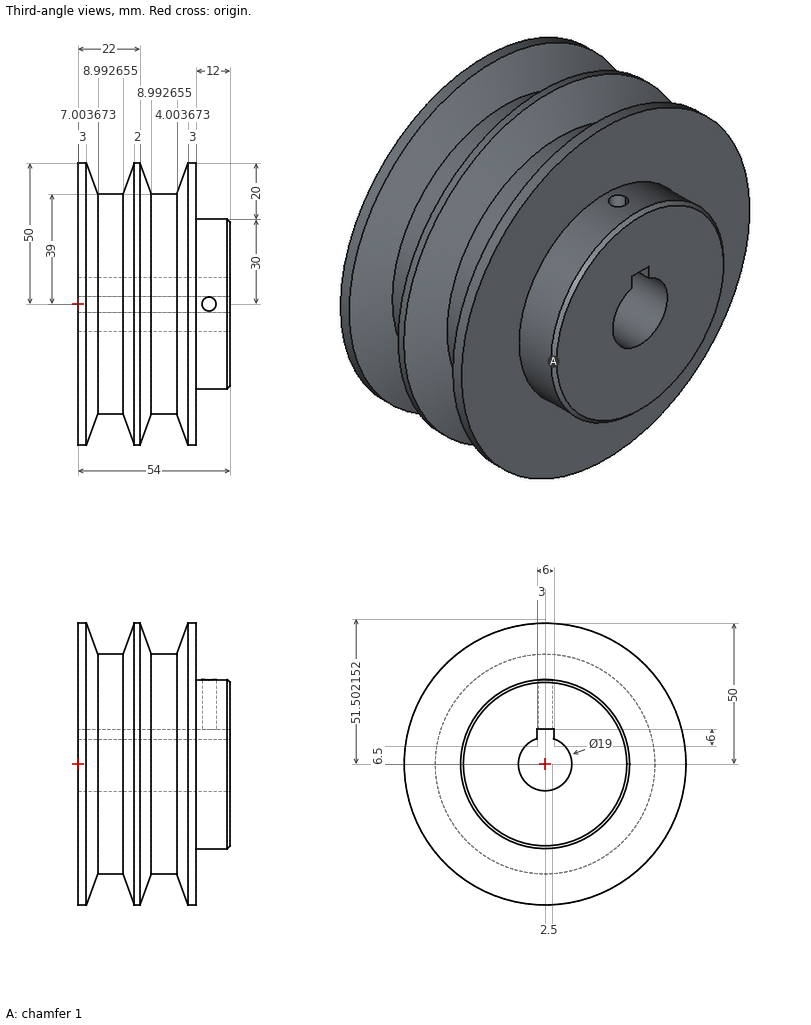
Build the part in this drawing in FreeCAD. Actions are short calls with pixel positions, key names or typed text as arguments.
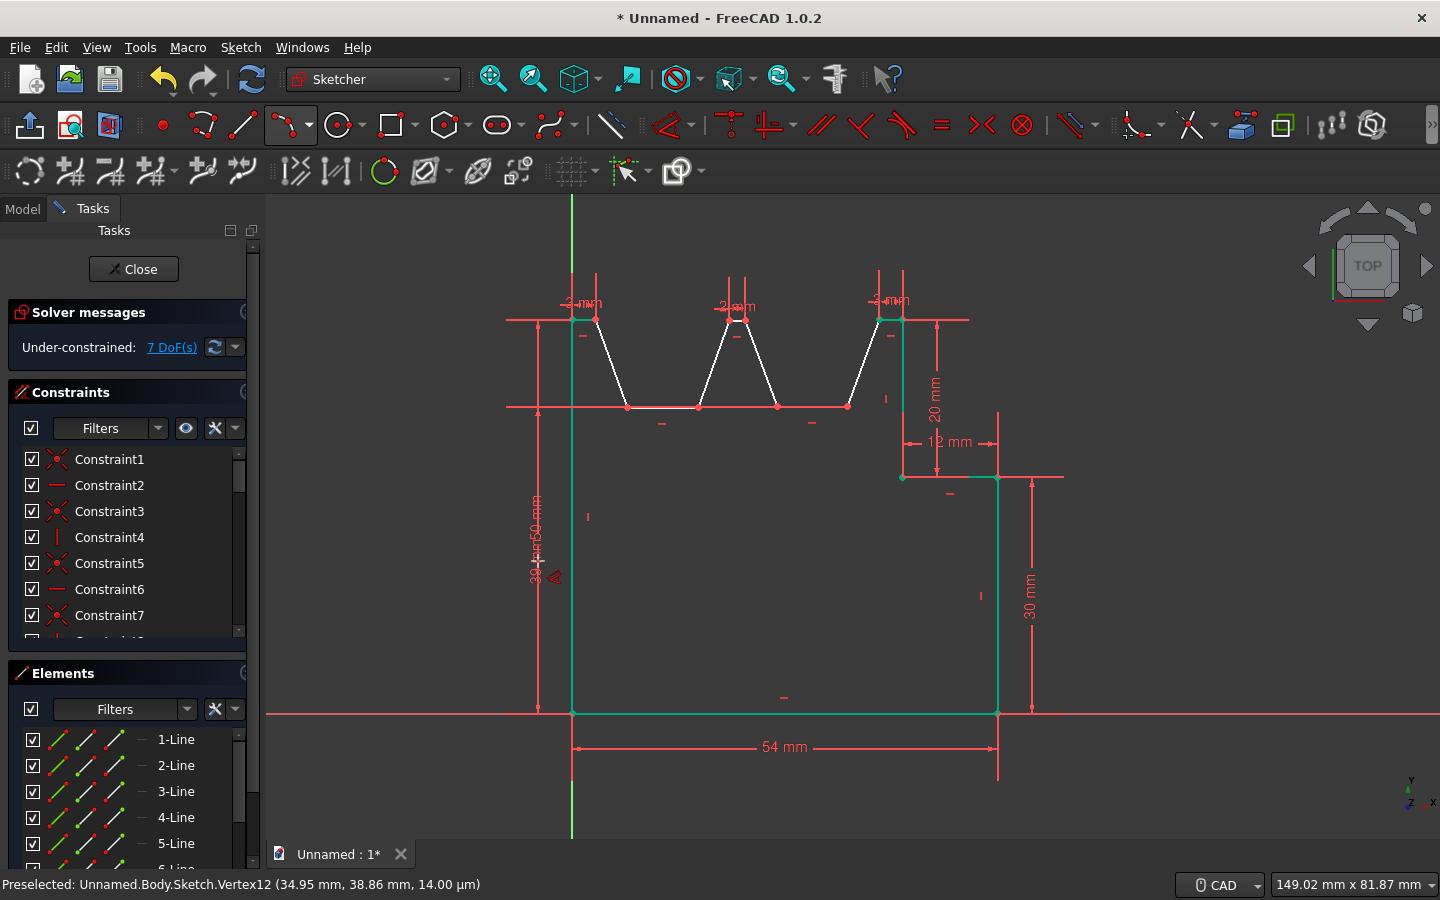
click(745, 321)
click(659, 748)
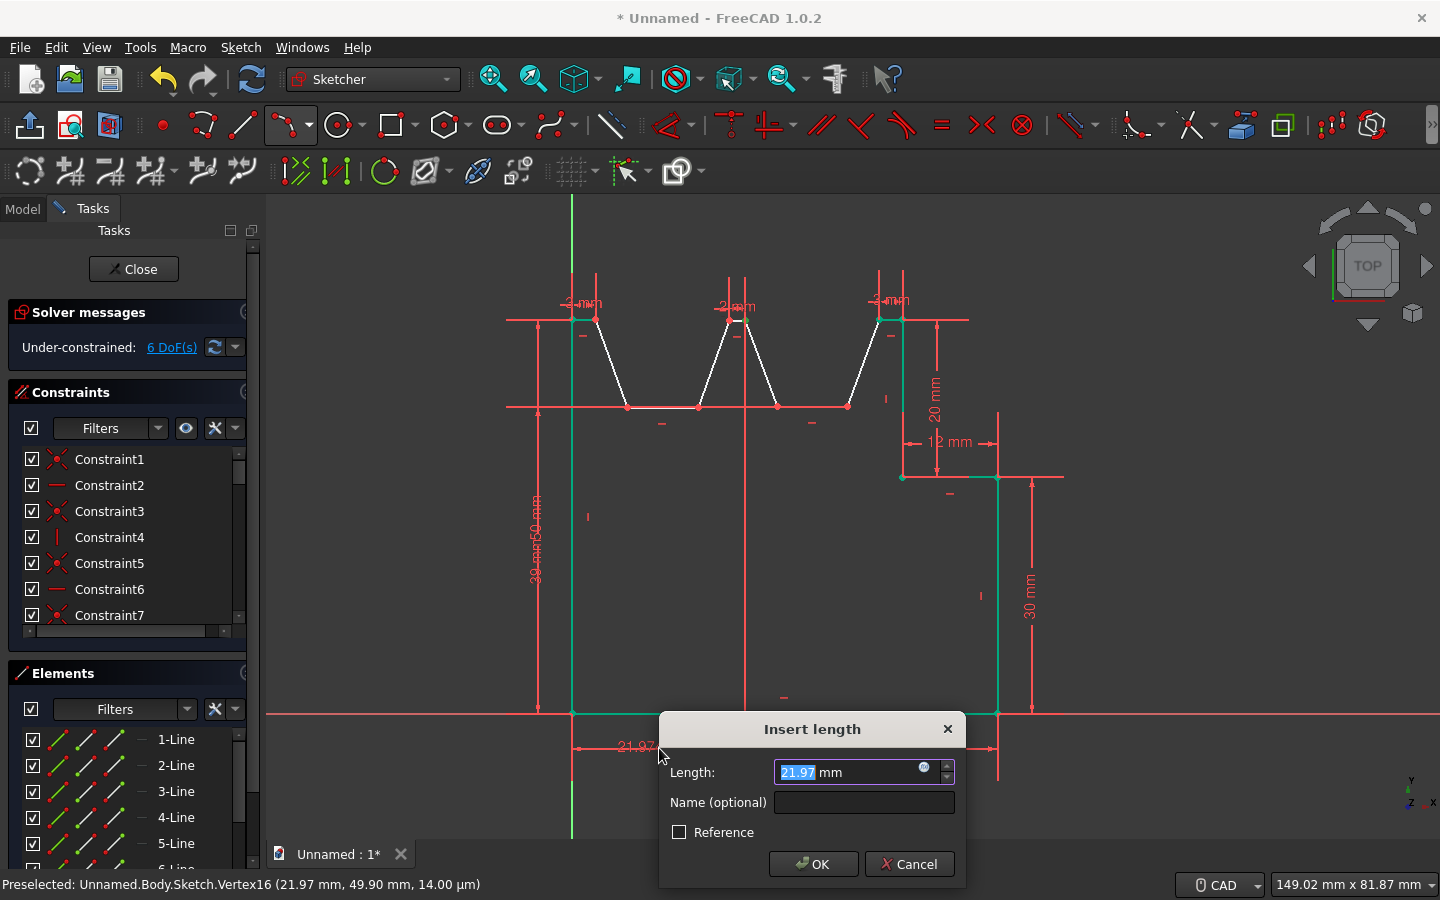
text(22)
key(Return)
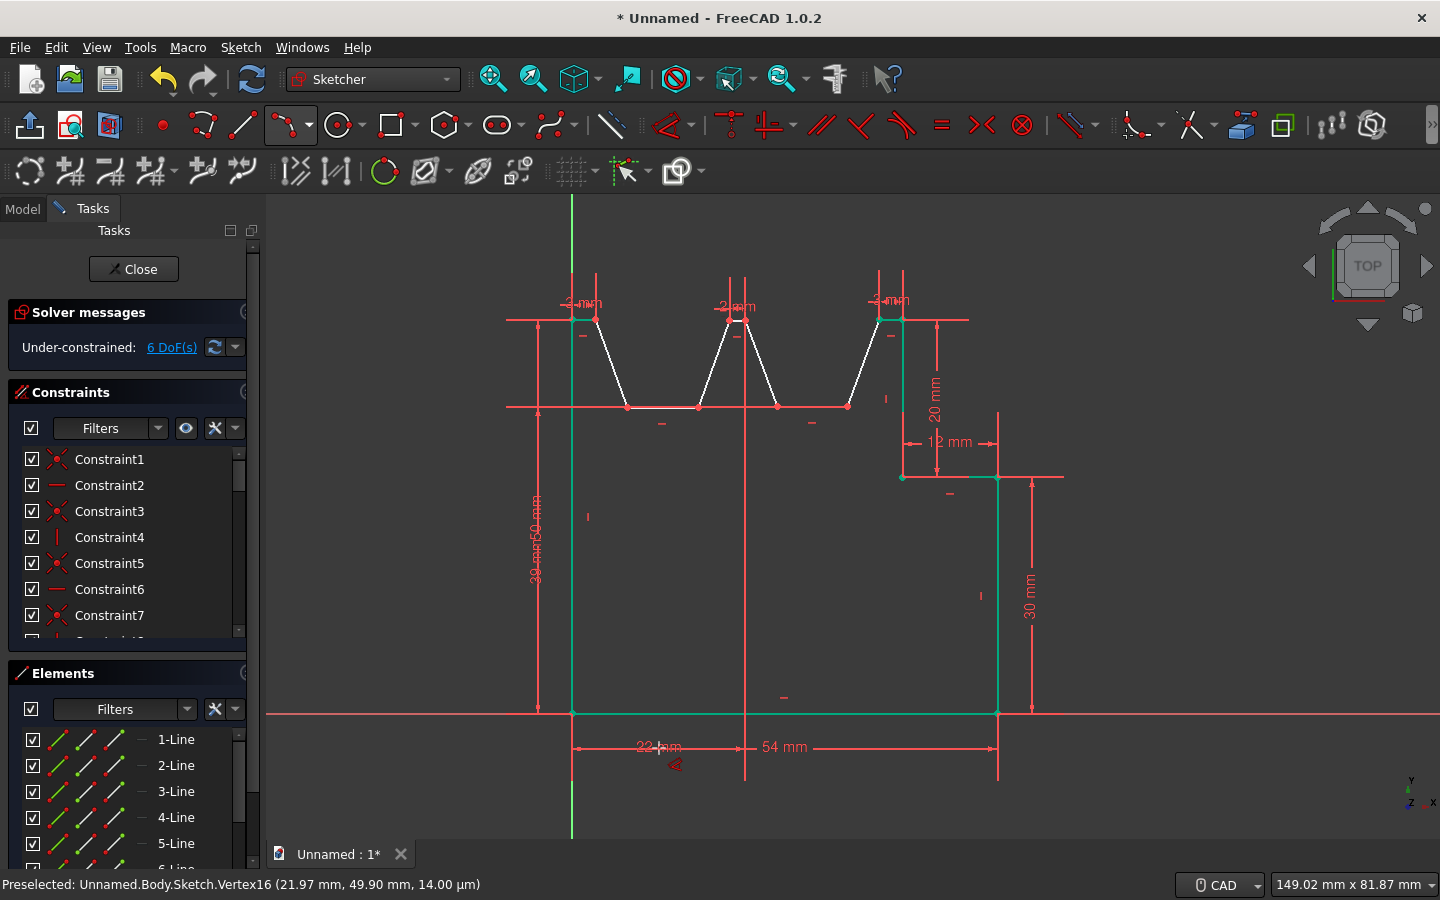
click(745, 321)
click(538, 427)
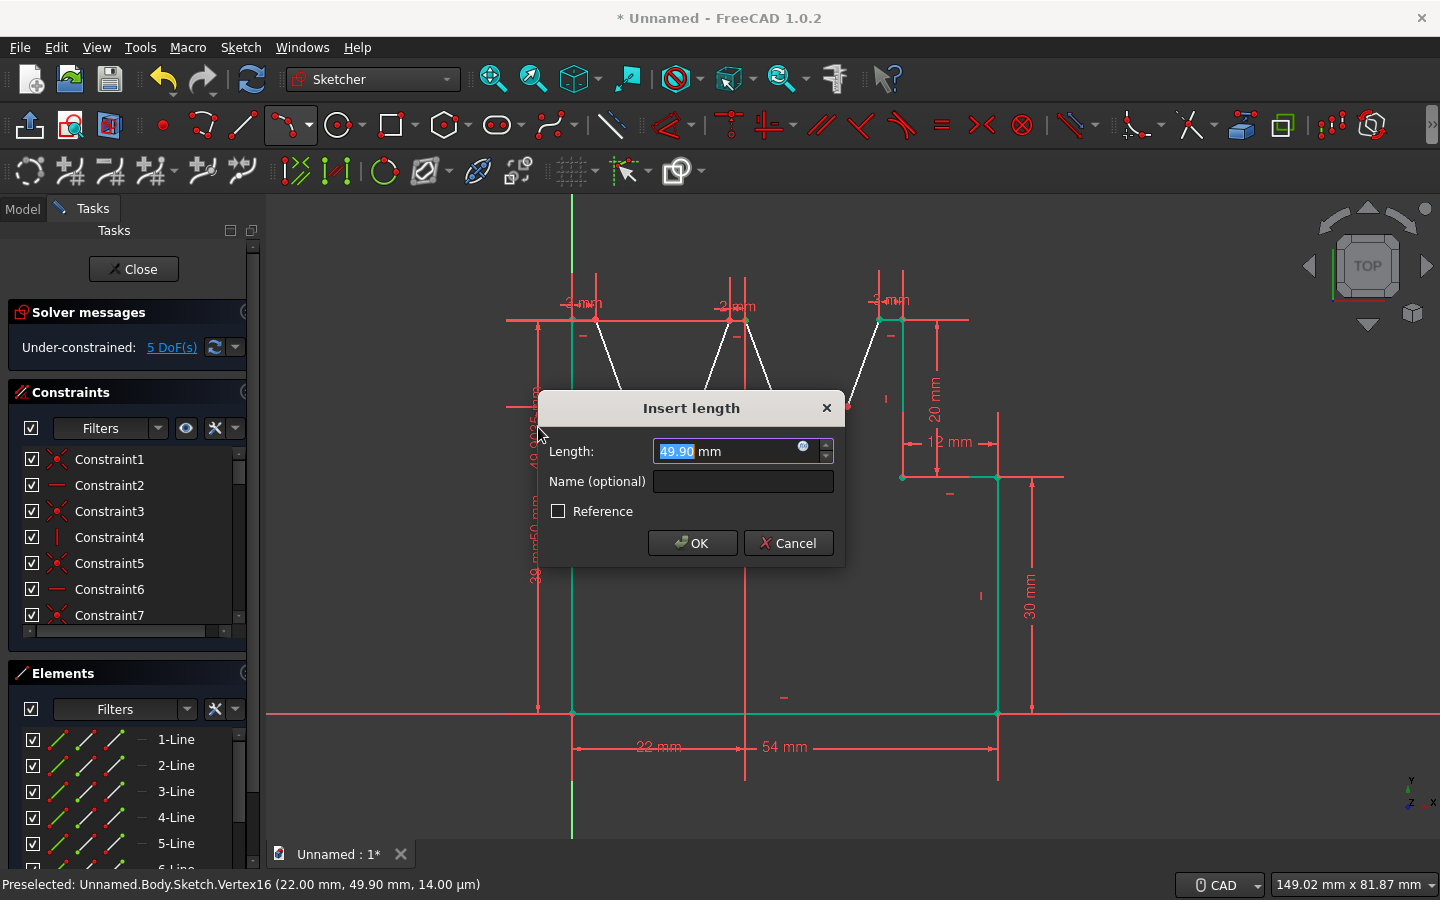
text(50)
key(Return)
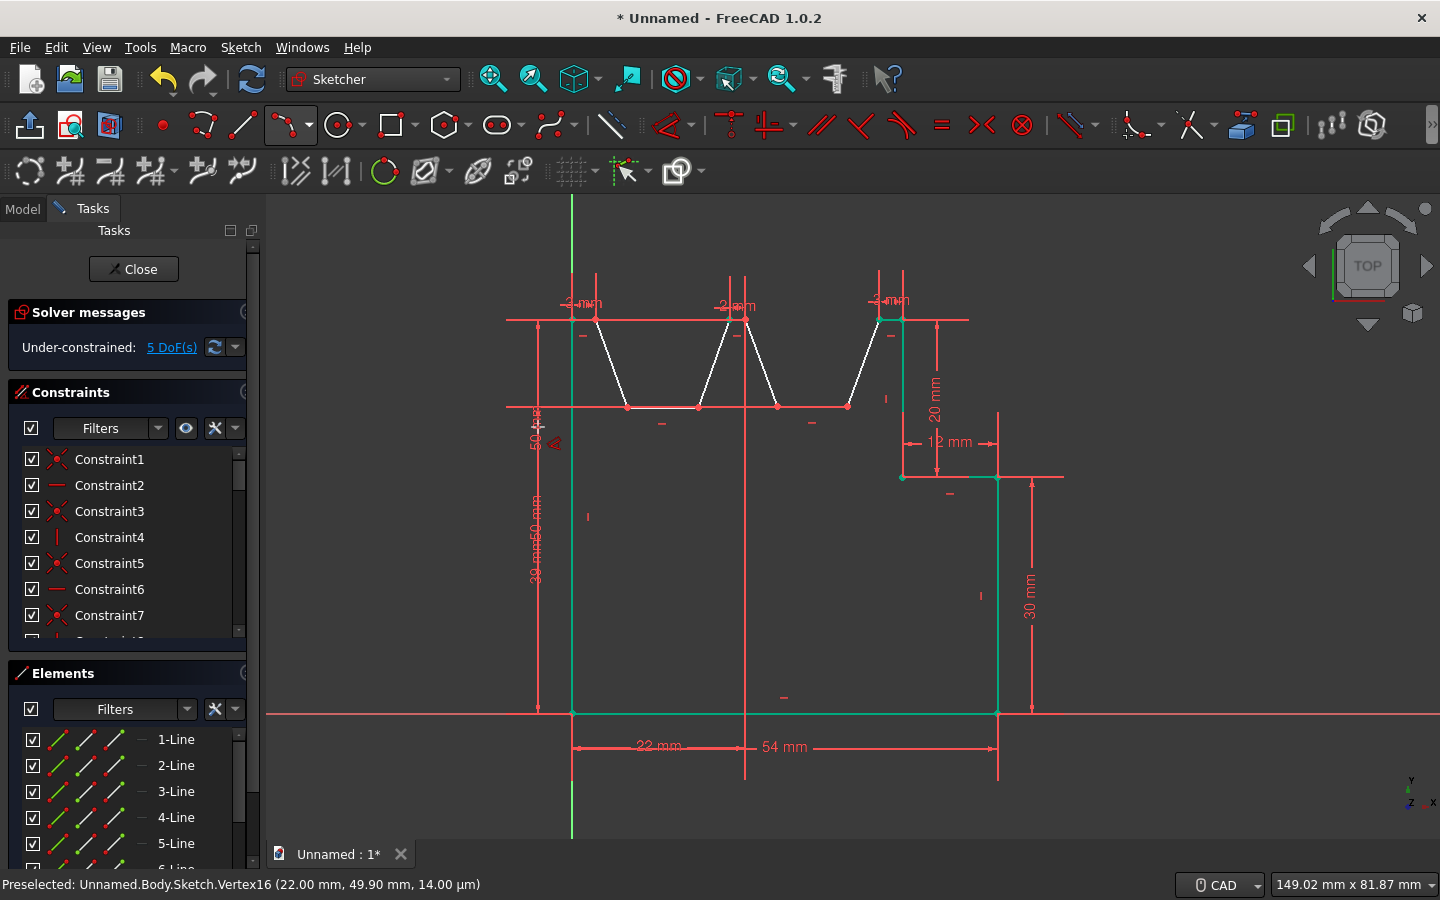
click(698, 408)
click(538, 490)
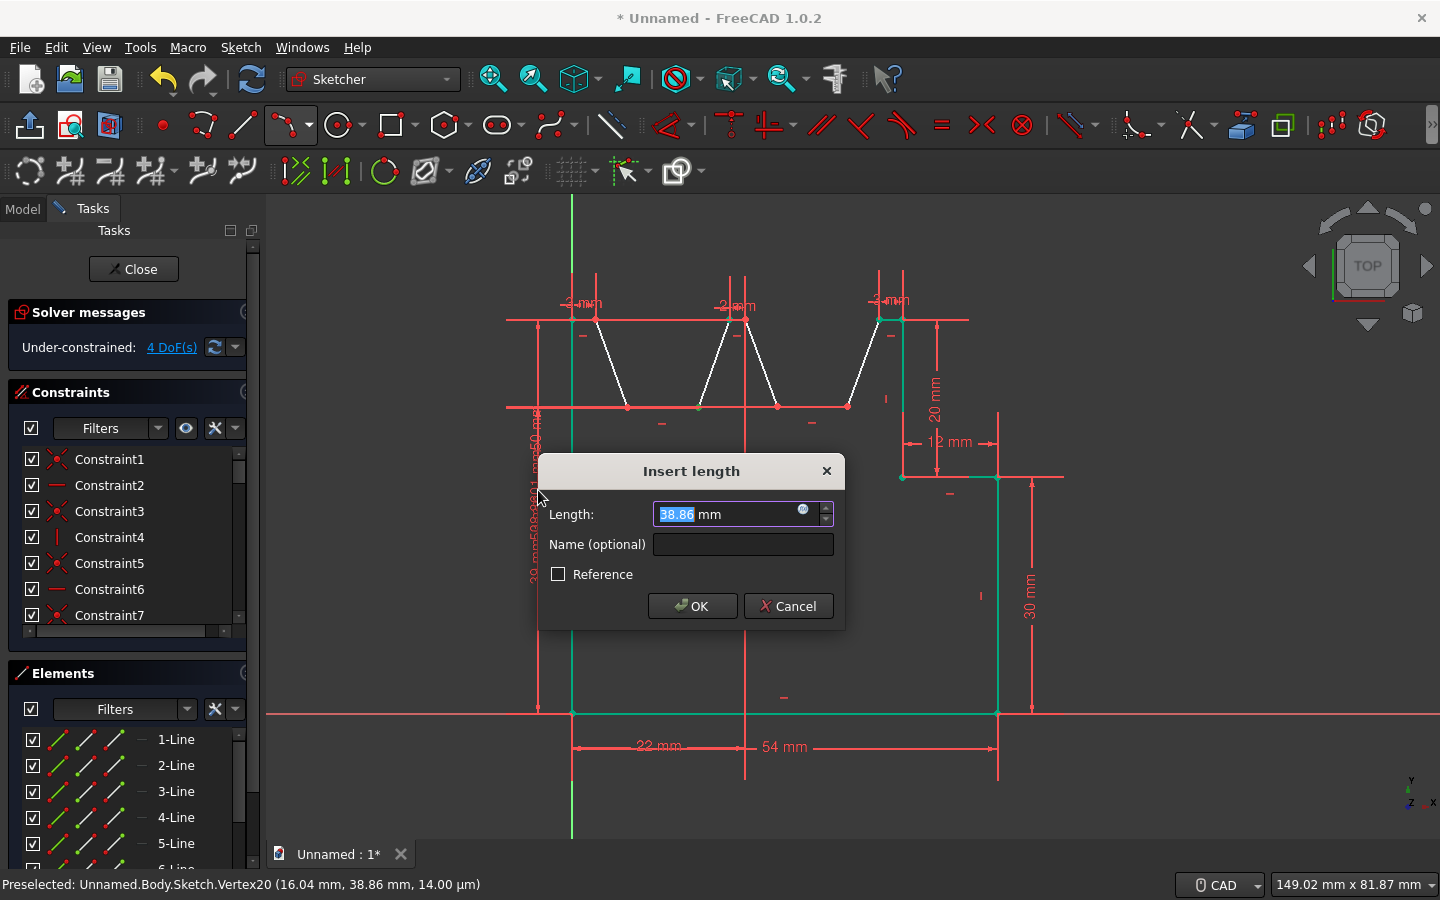
text(39)
key(Return)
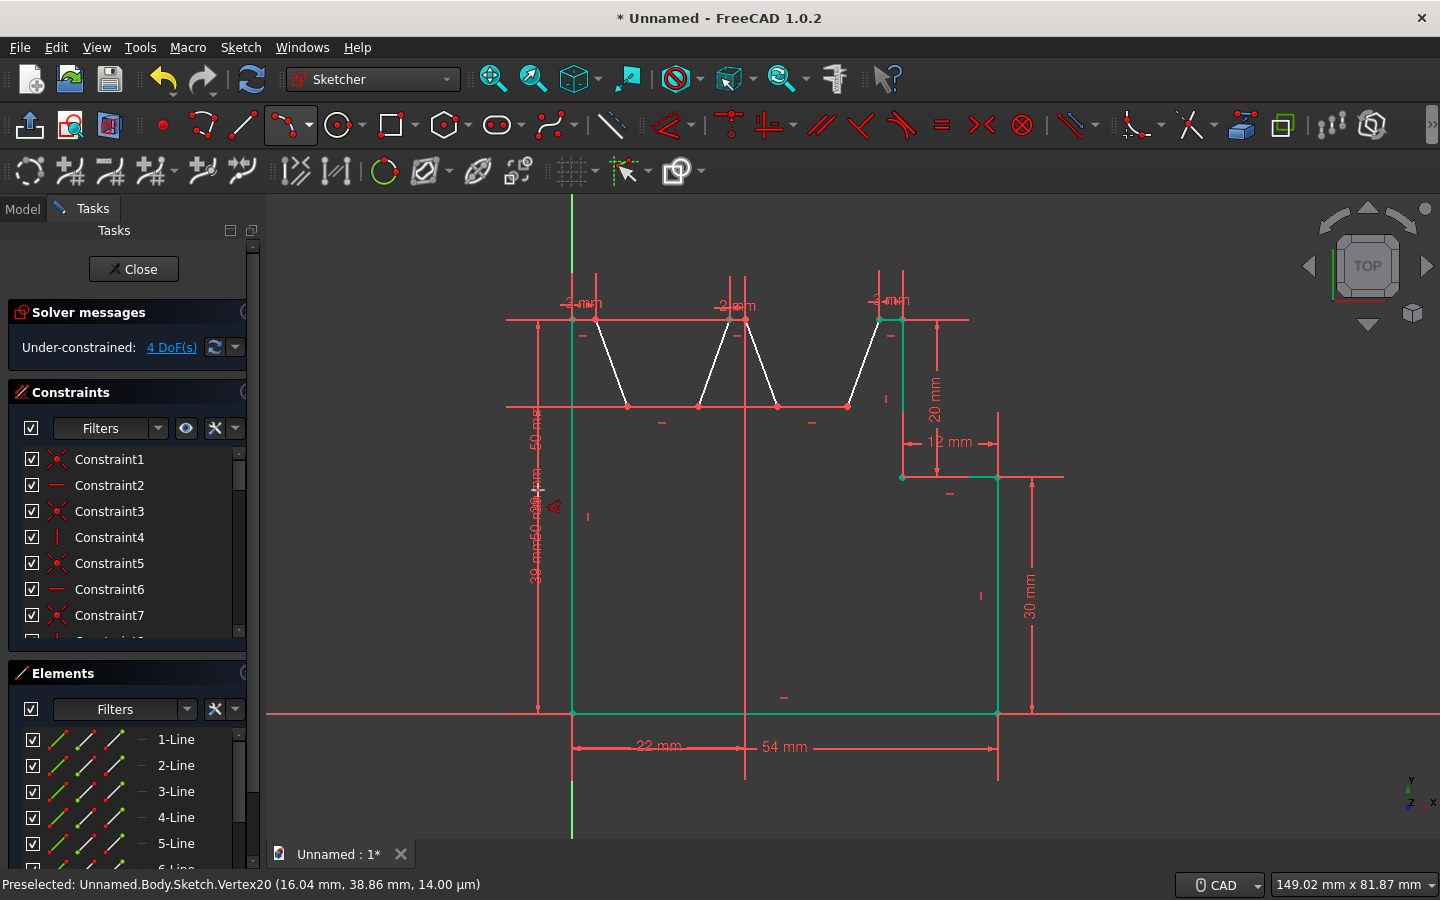
click(826, 407)
click(812, 373)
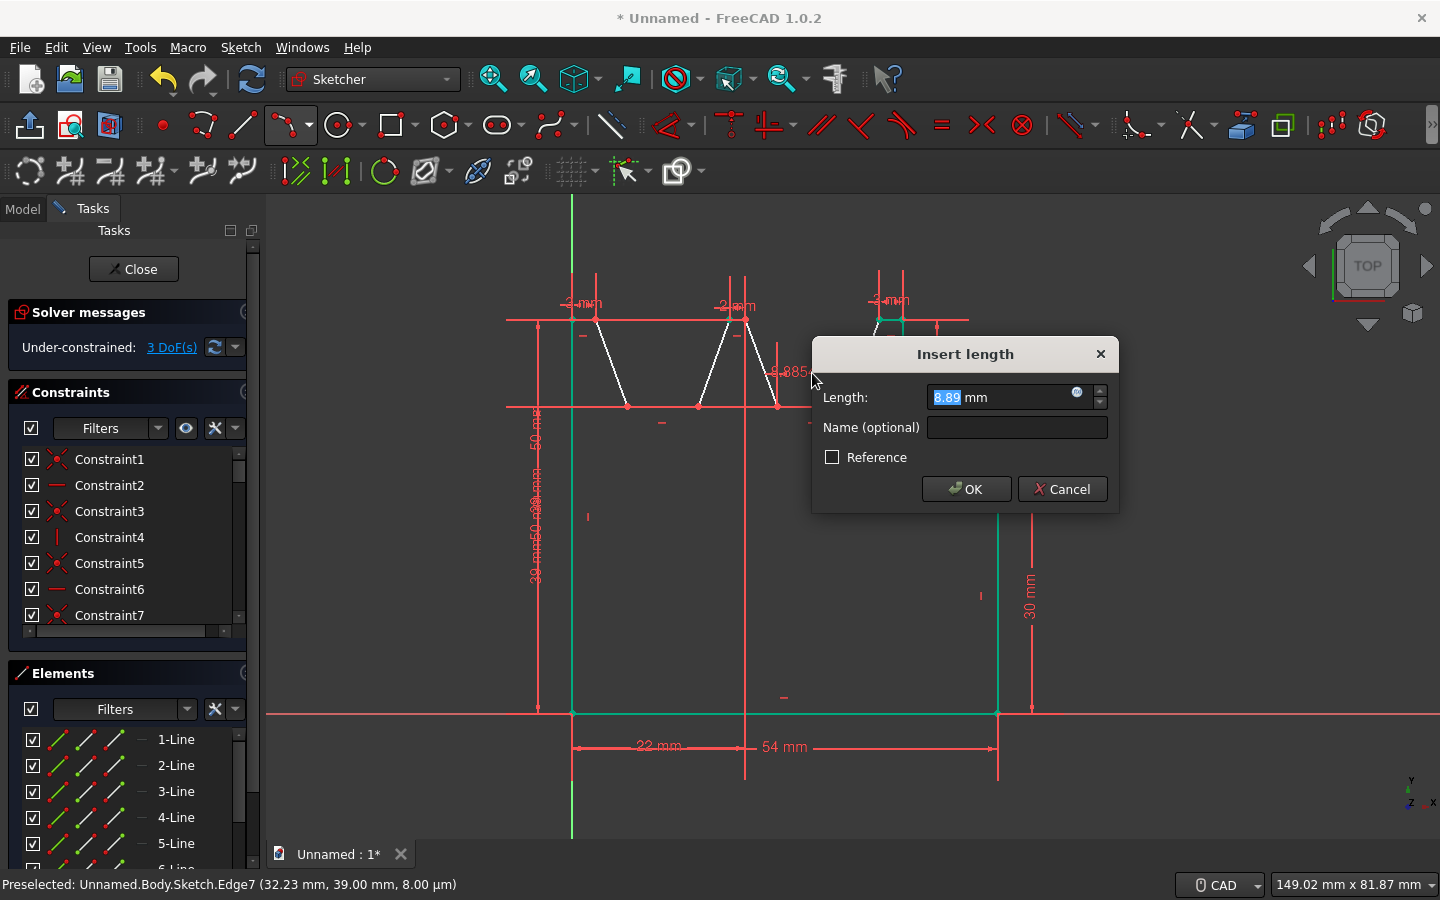
text(8.992655)
key(Return)